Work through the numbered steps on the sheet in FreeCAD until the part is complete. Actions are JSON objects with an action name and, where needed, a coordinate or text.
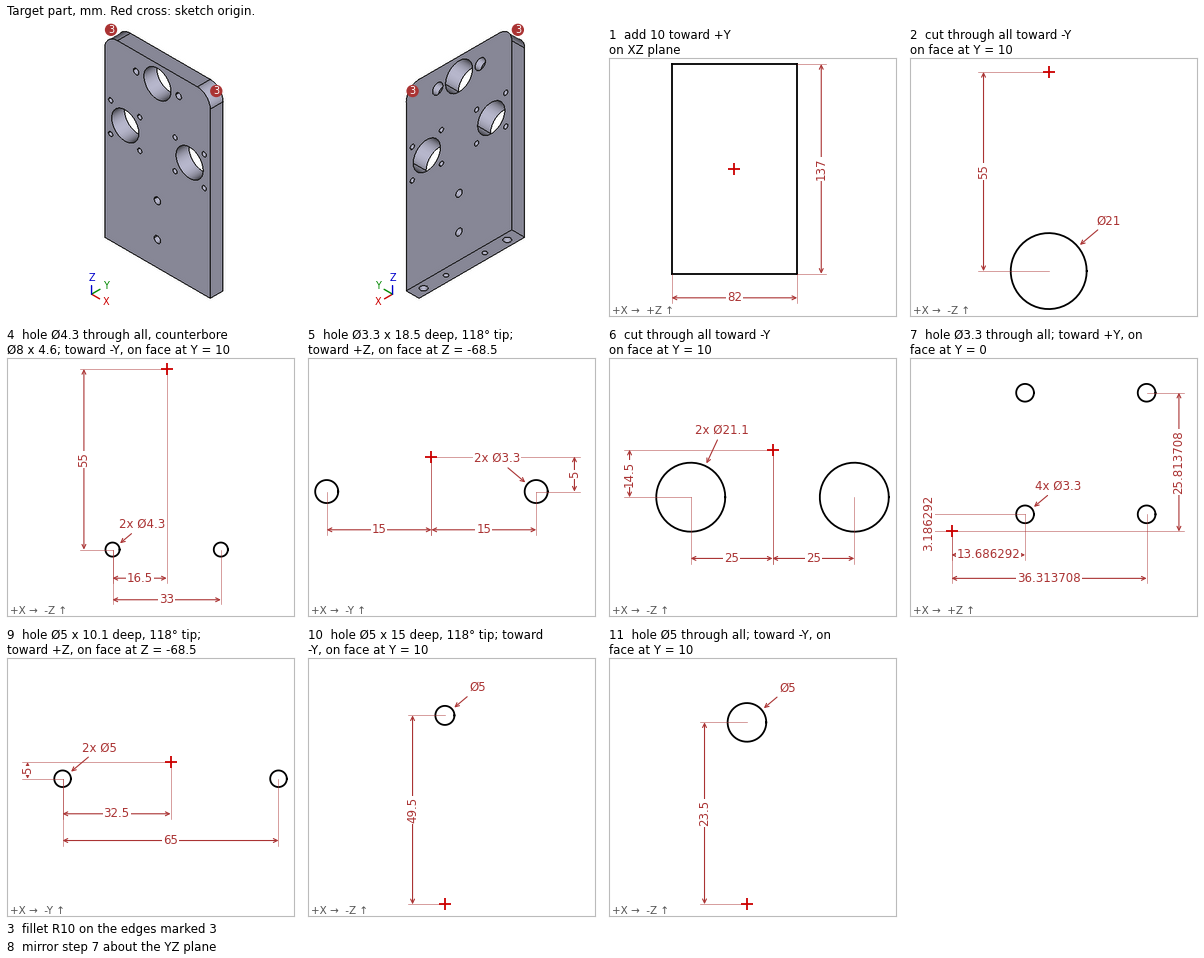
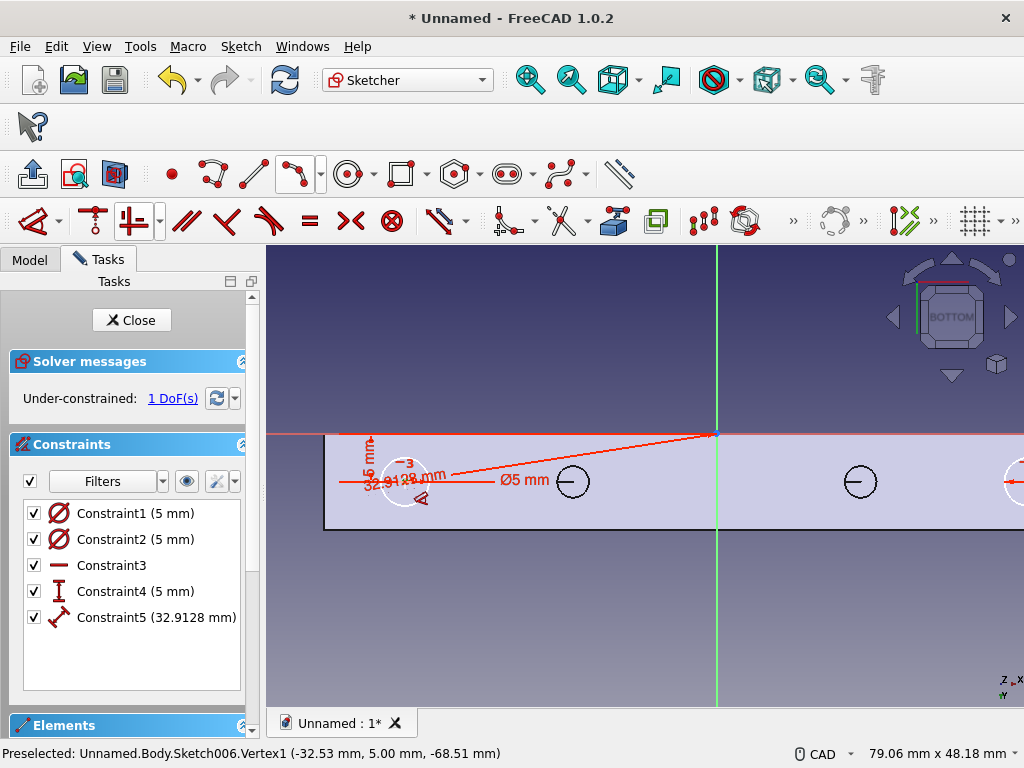
{"action": "scroll", "coordinate": [406, 483], "scroll_direction": "down", "scroll_amount": 3}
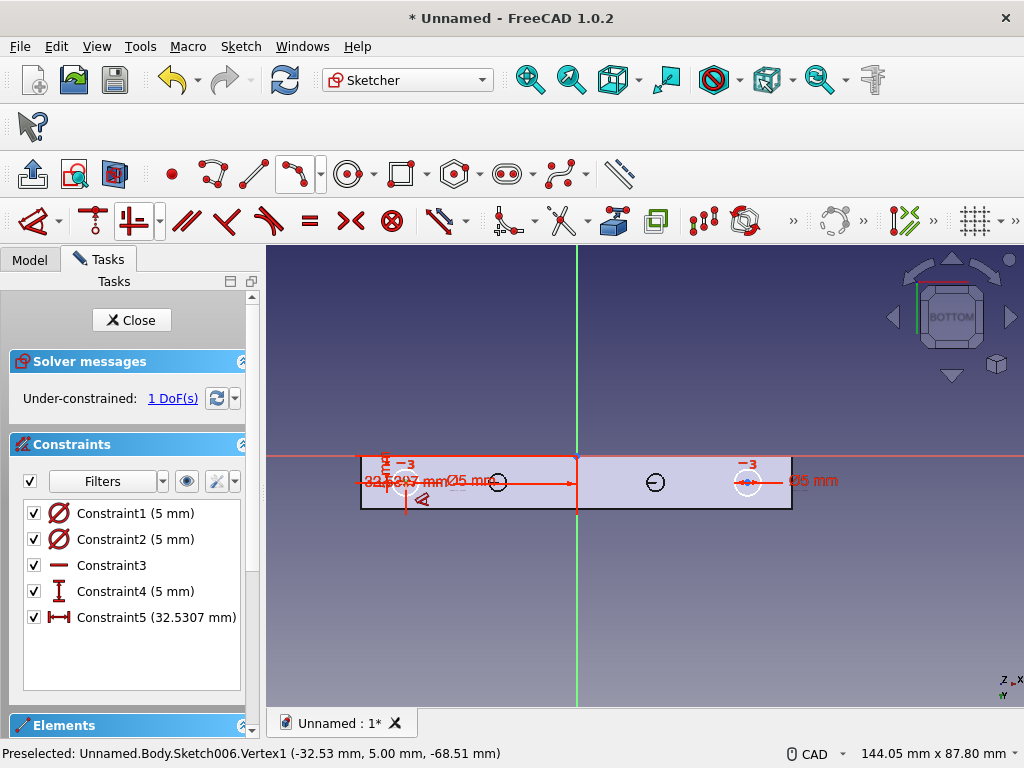
{"action": "left_click", "coordinate": [748, 483]}
{"action": "left_click", "coordinate": [498, 517]}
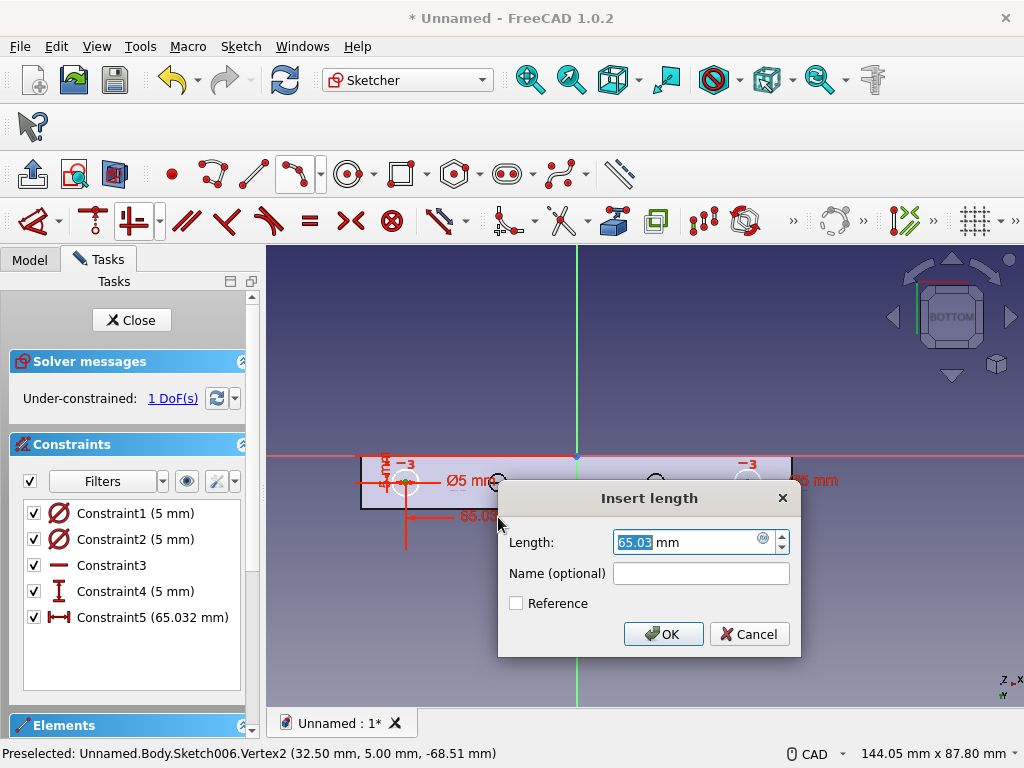
{"action": "type", "text": "65"}
{"action": "key", "text": "Return"}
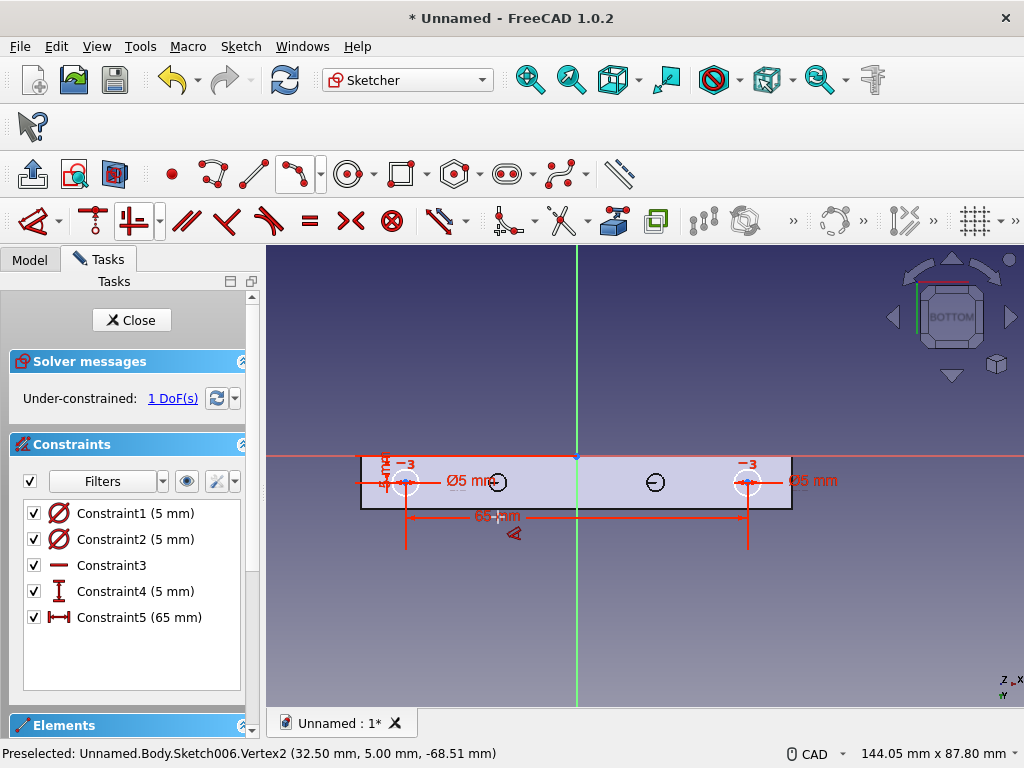
{"action": "left_click", "coordinate": [406, 483]}
{"action": "left_click", "coordinate": [491, 422]}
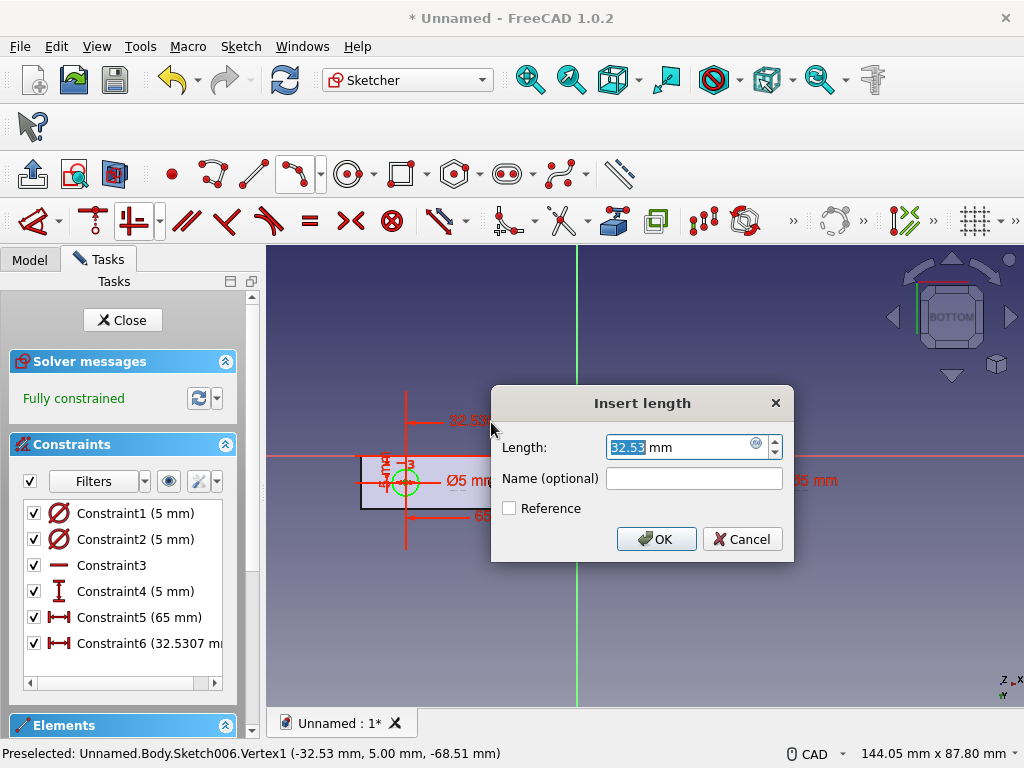
{"action": "type", "text": "32.5"}
{"action": "key", "text": "Return"}
{"action": "key", "text": "Escape"}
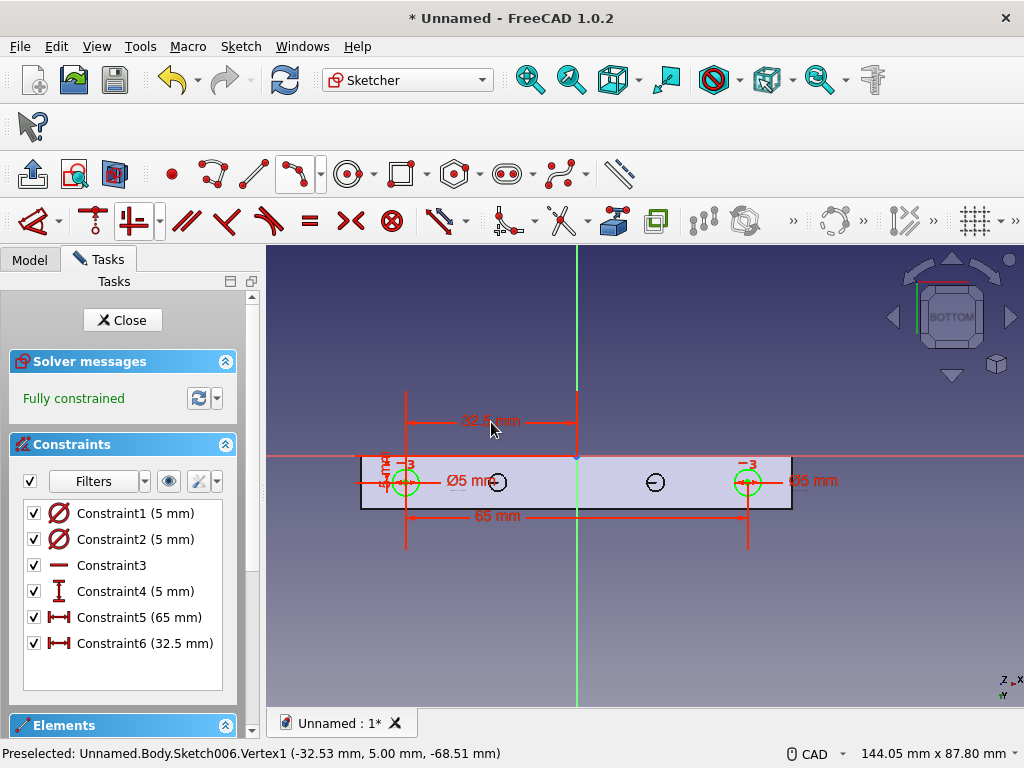
{"action": "left_click", "coordinate": [123, 320]}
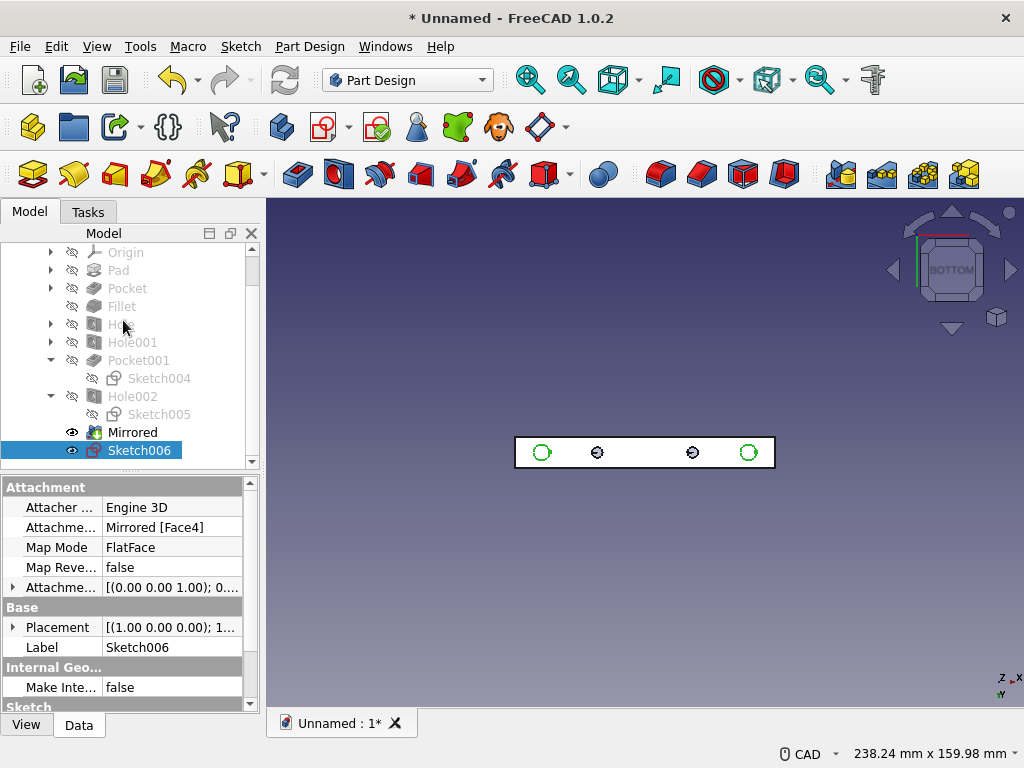
{"action": "left_click", "coordinate": [339, 174]}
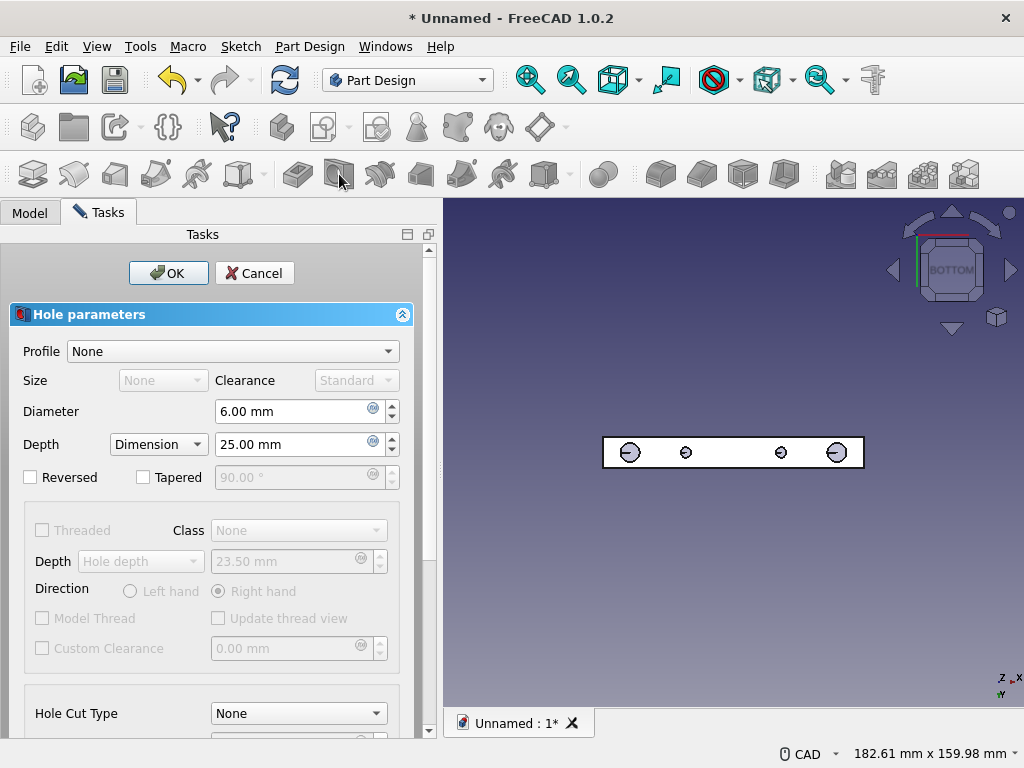
{"action": "triple_click", "coordinate": [300, 412]}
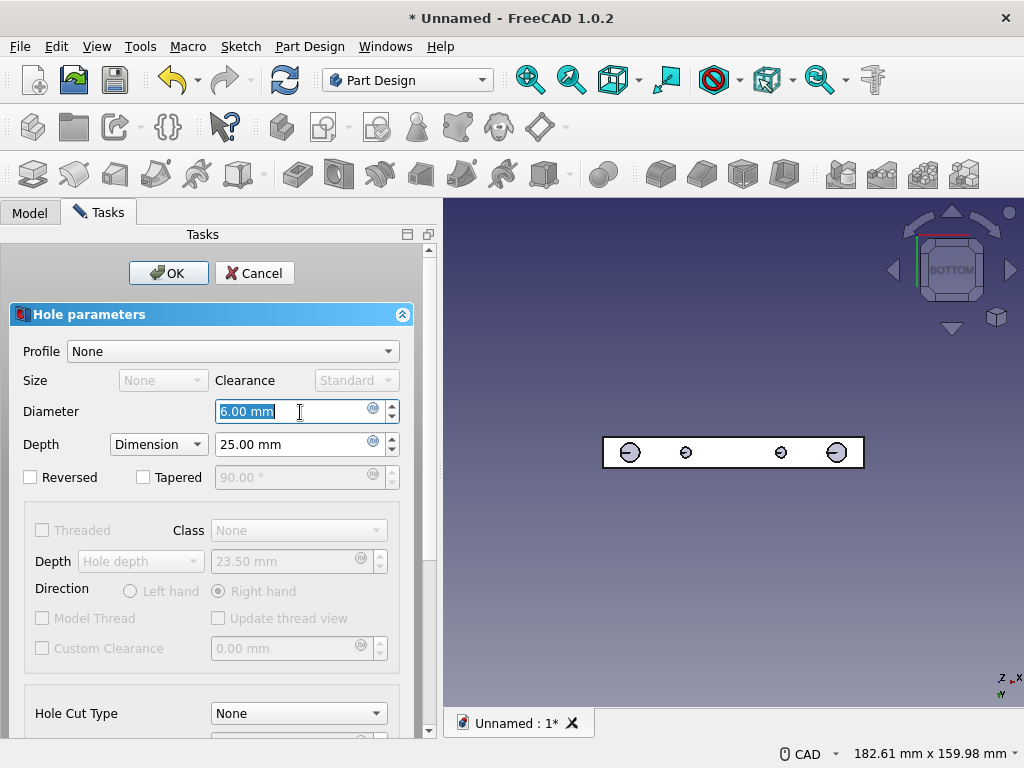
{"action": "type", "text": "5"}
{"action": "key", "text": "Tab"}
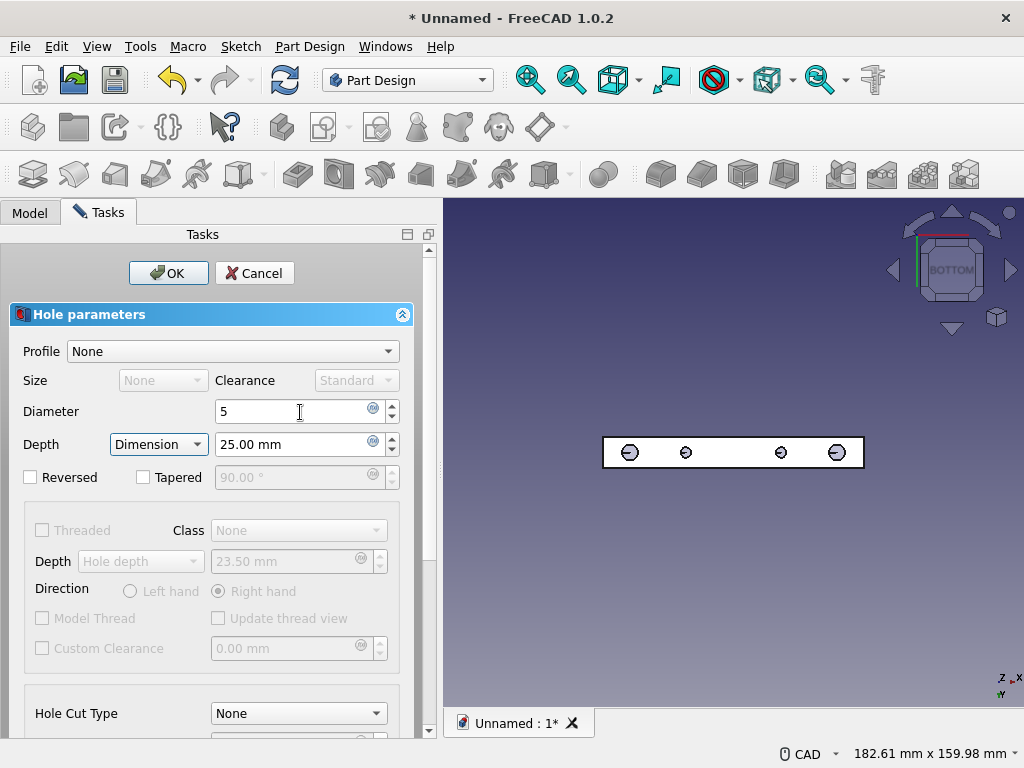
{"action": "triple_click", "coordinate": [300, 444]}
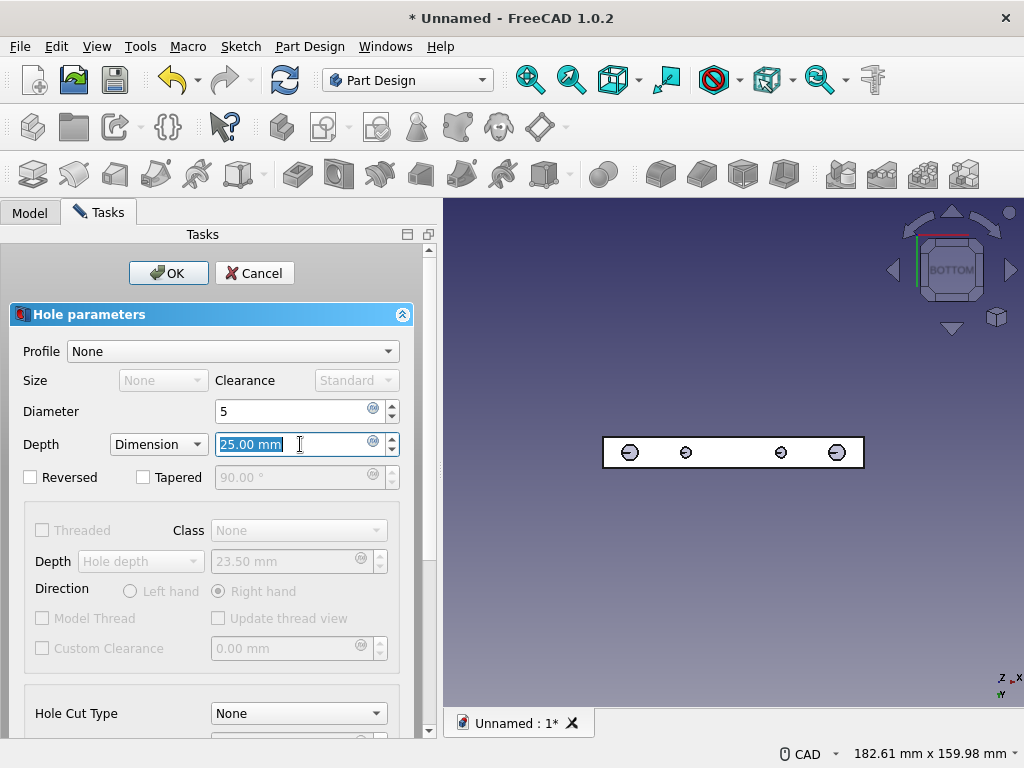
{"action": "type", "text": "10.1"}
{"action": "key", "text": "Tab"}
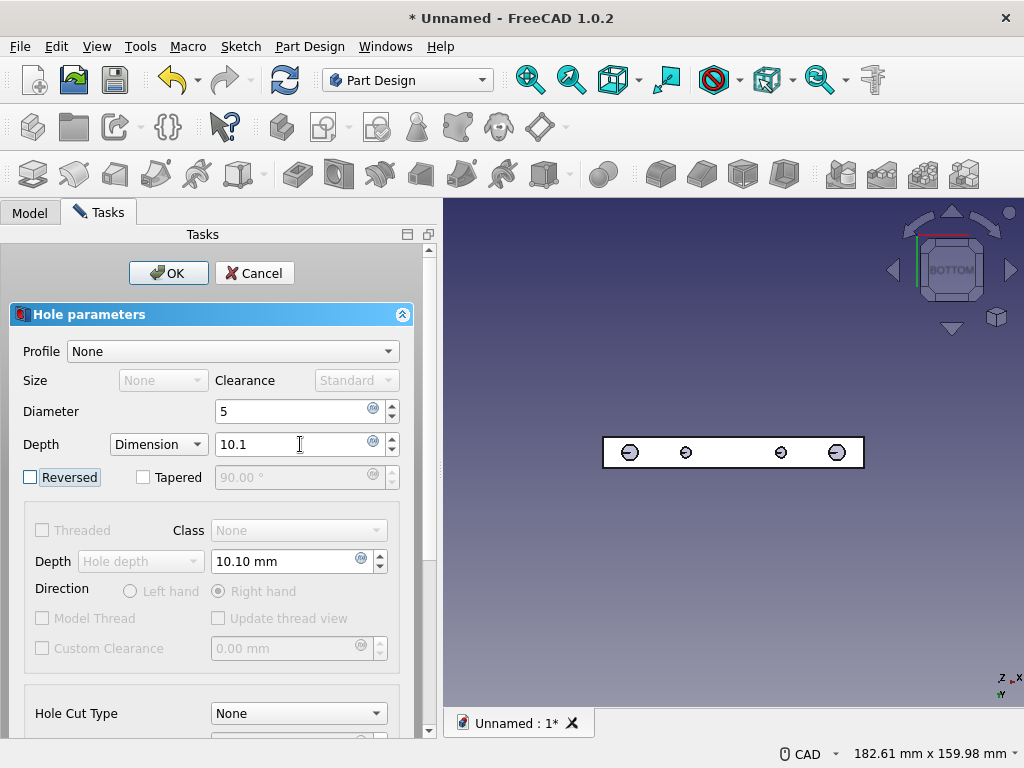
{"action": "left_click", "coordinate": [169, 273]}